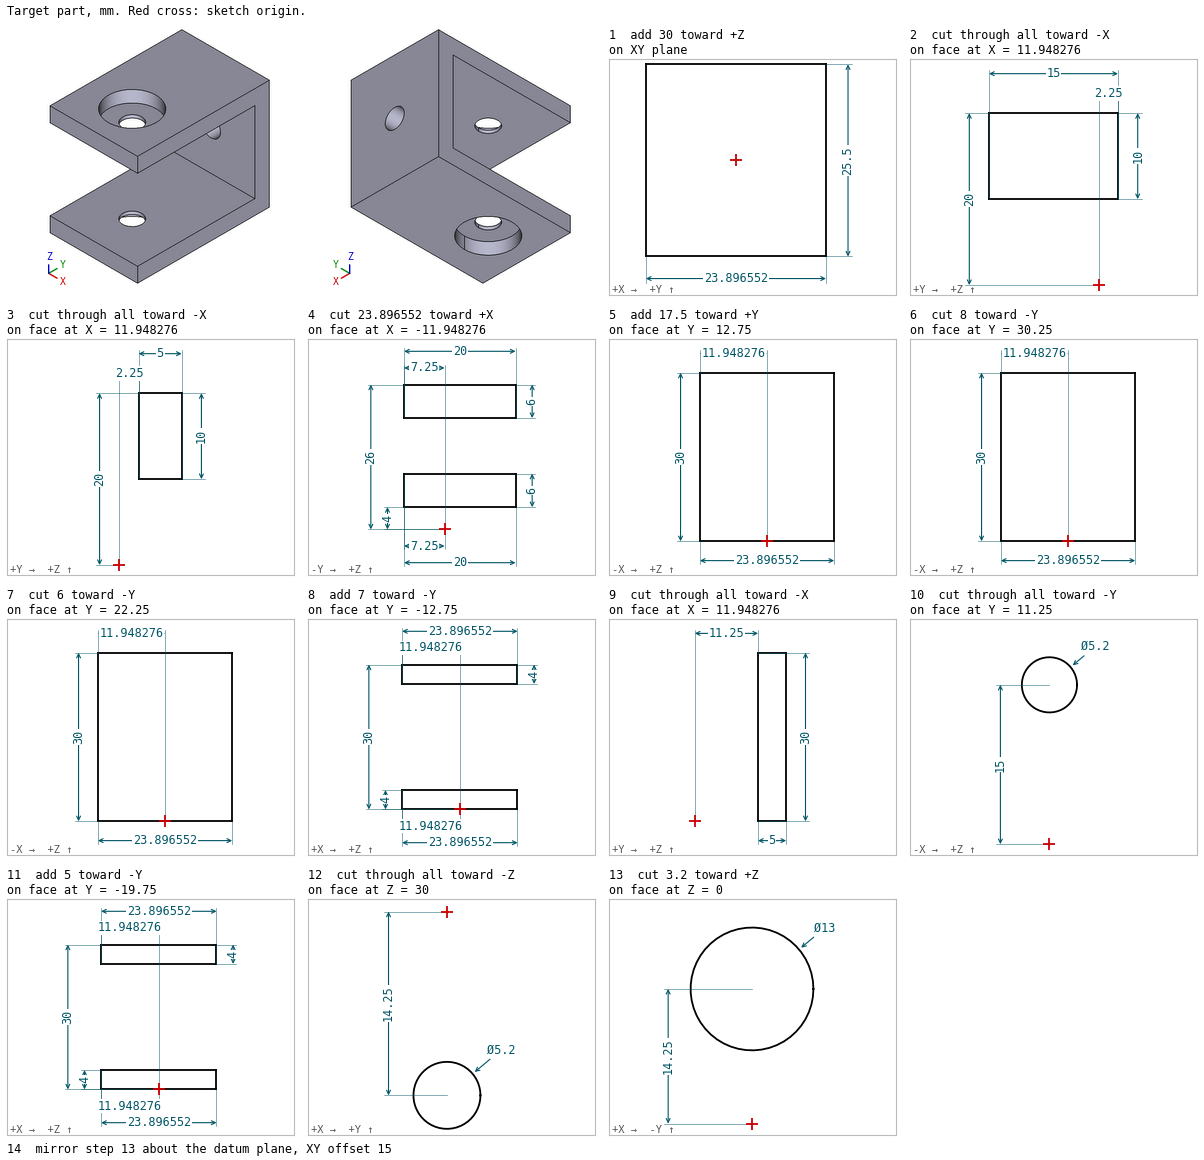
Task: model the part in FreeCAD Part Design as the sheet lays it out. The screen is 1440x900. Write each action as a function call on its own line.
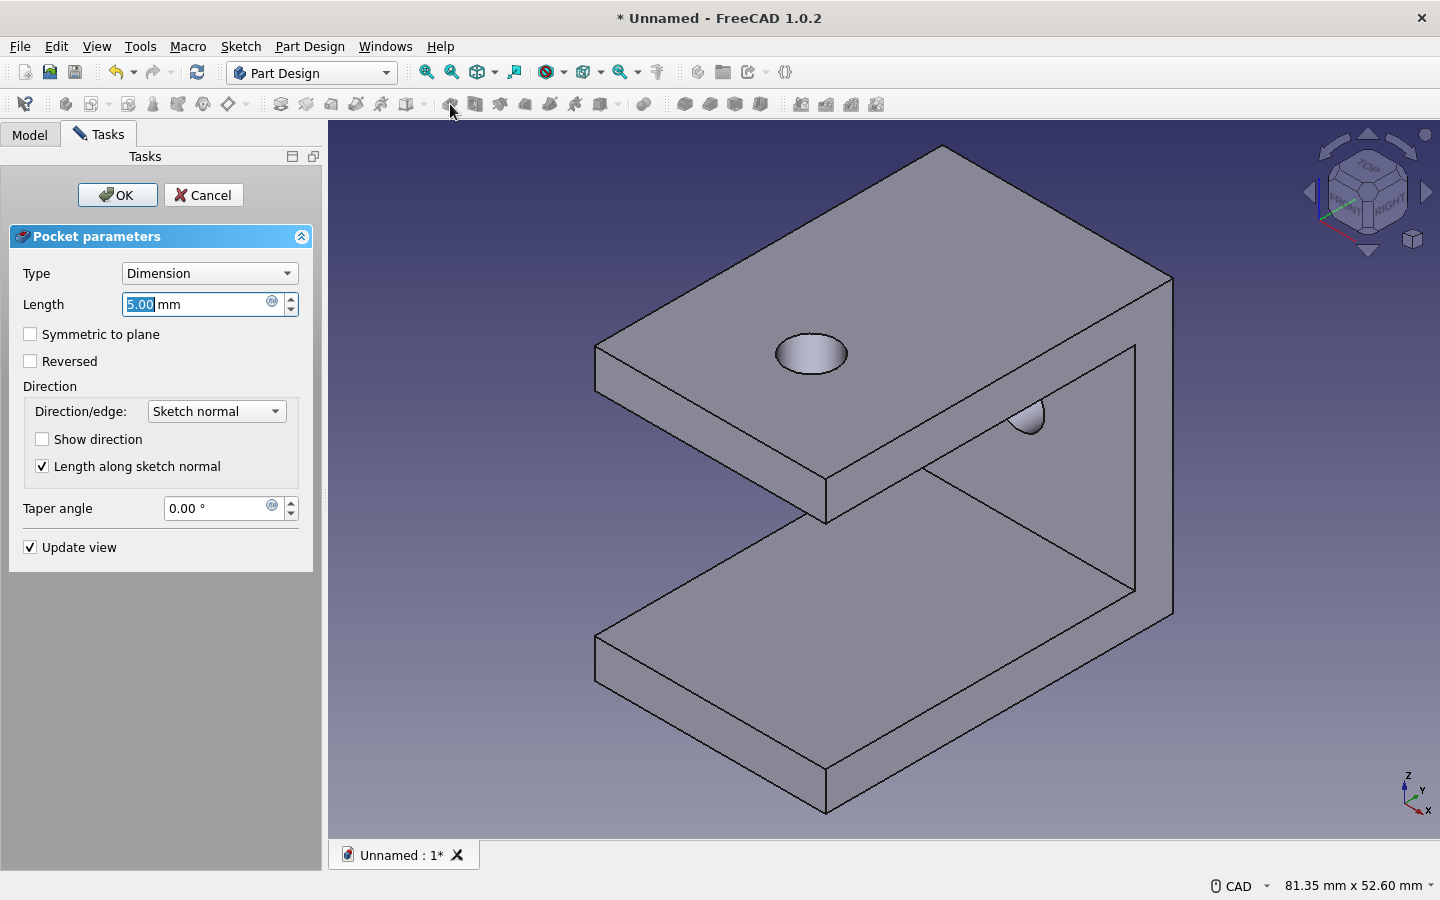
click(210, 274)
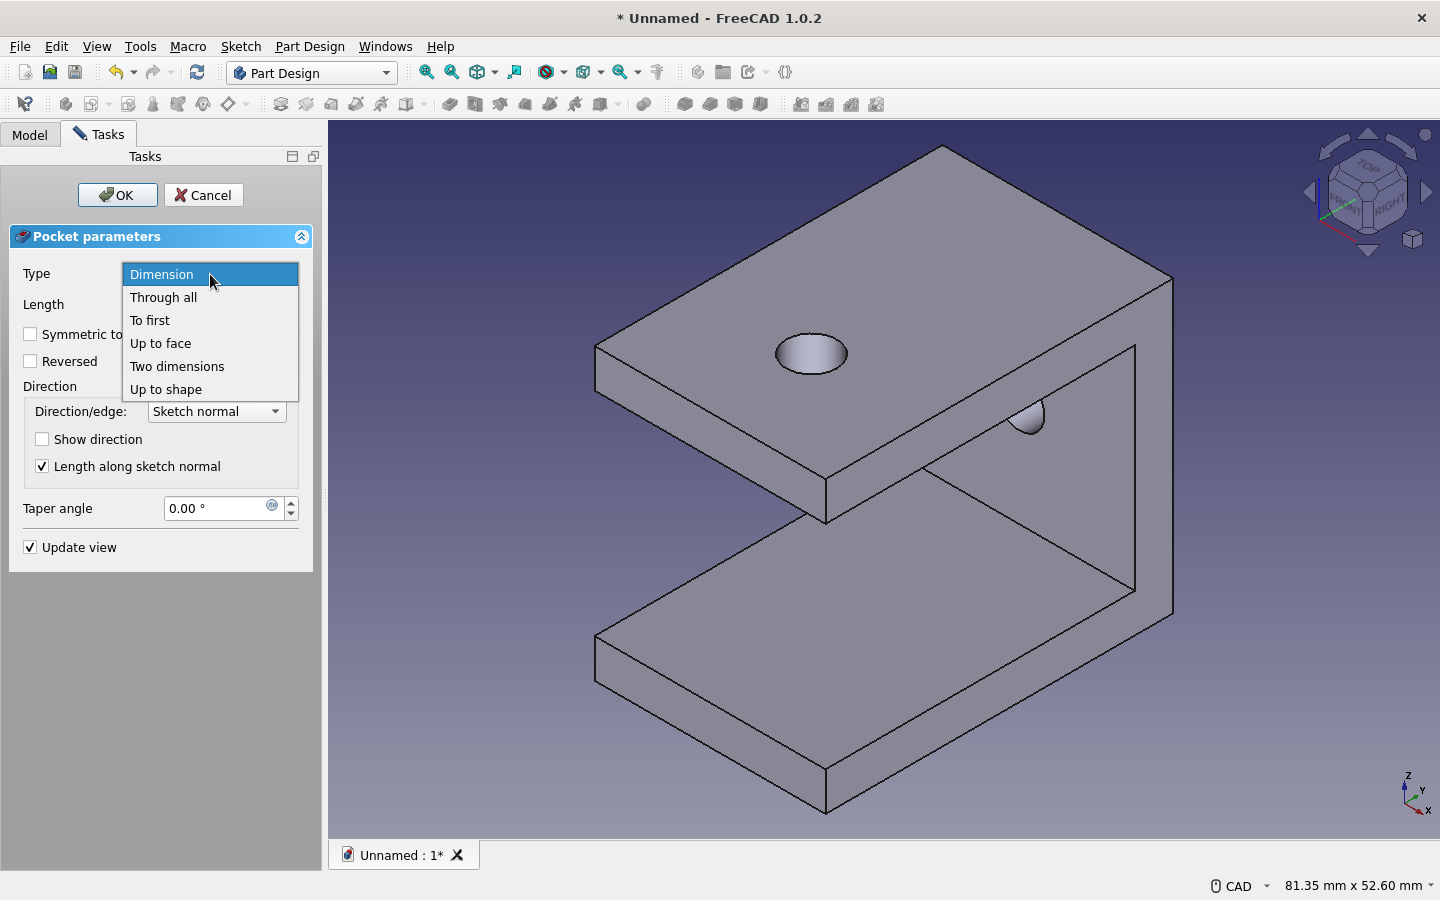
click(208, 298)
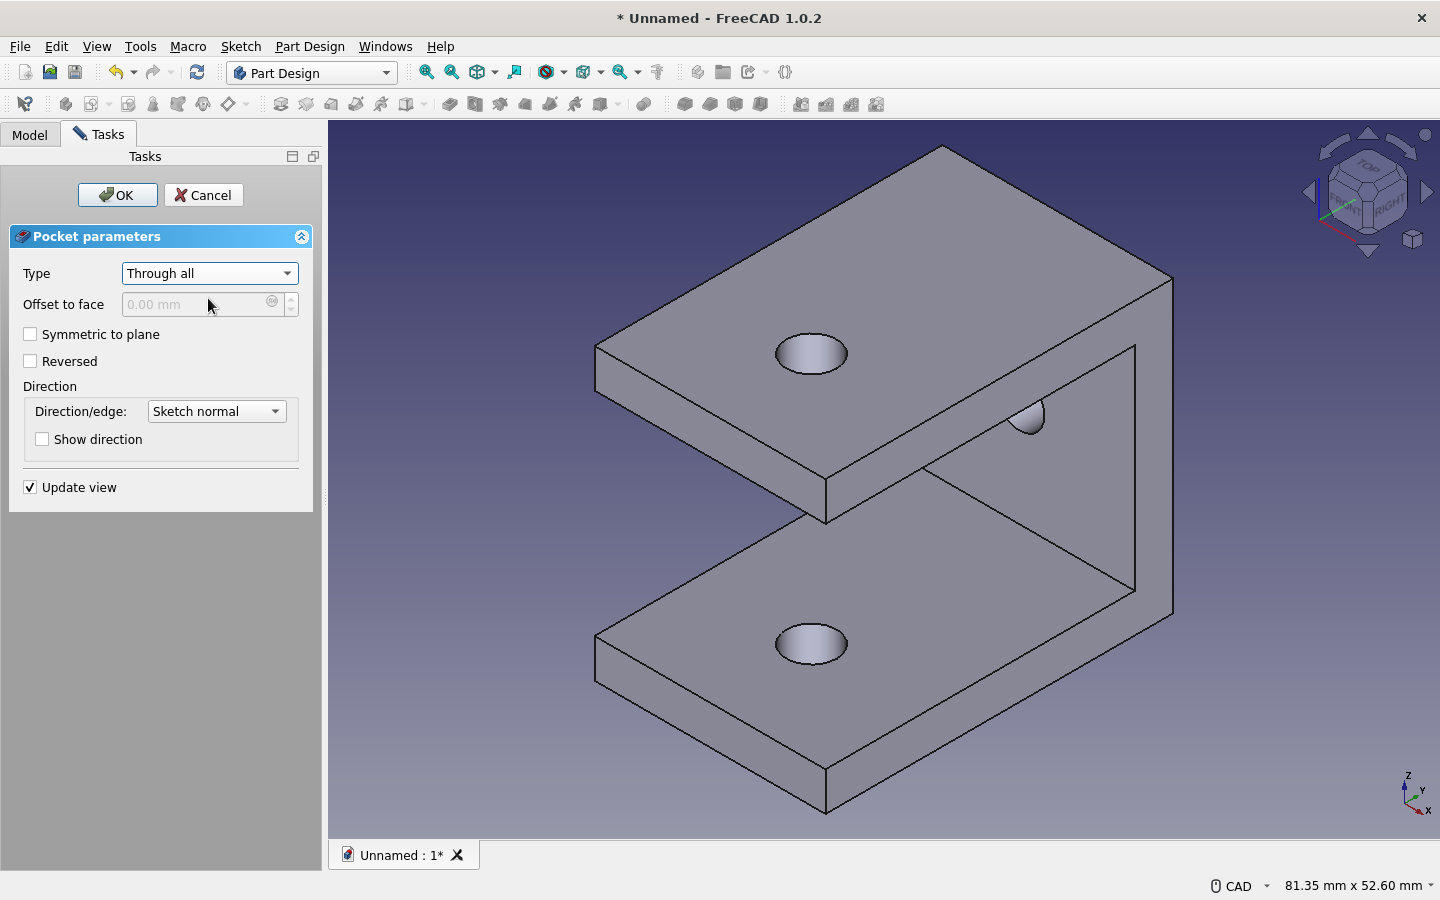
click(118, 195)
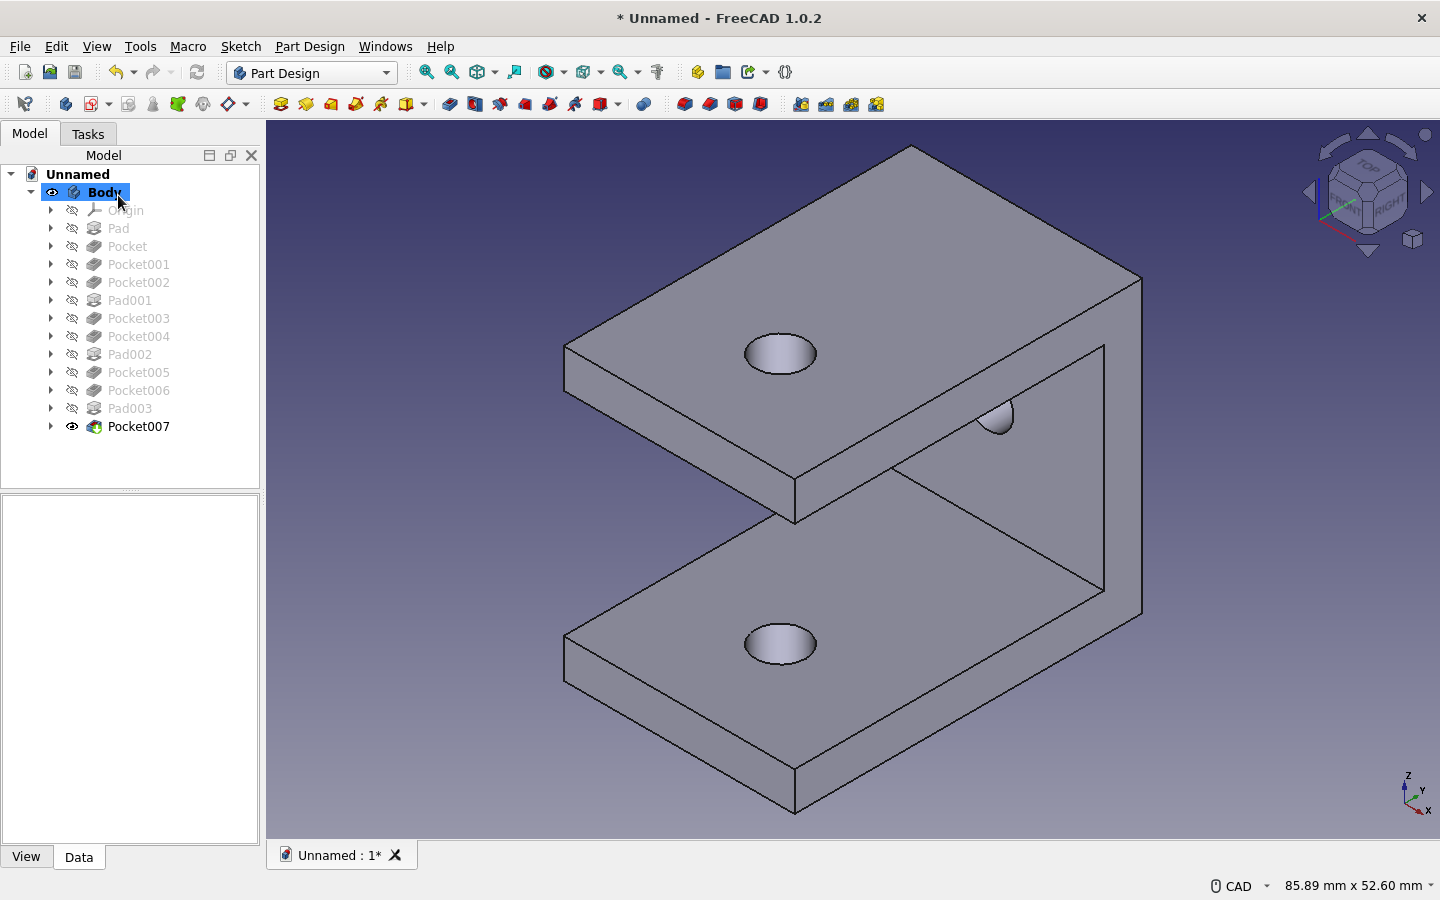
key(5)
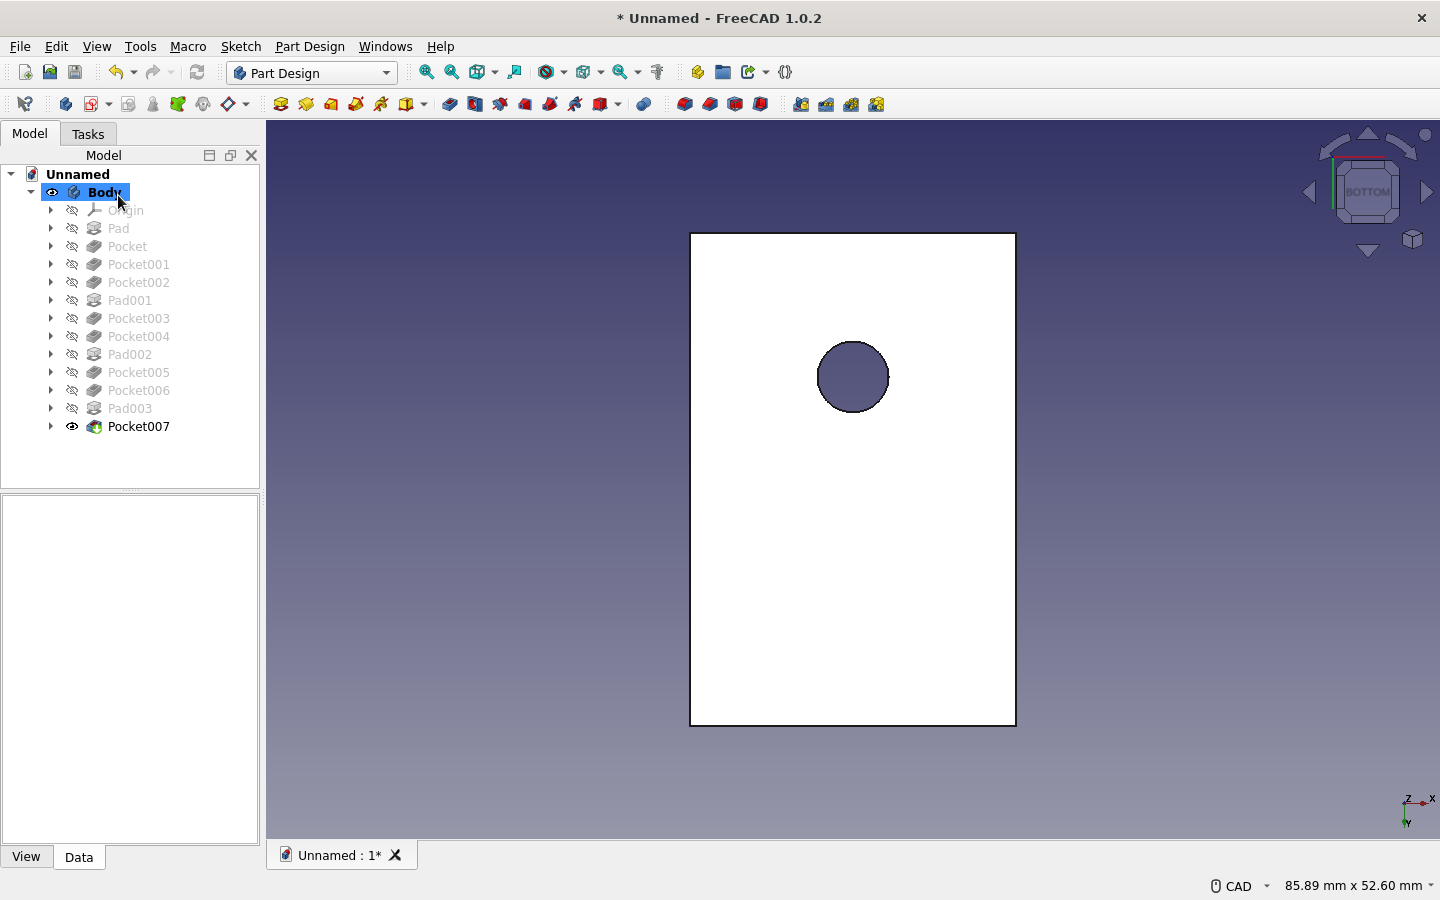
click(853, 549)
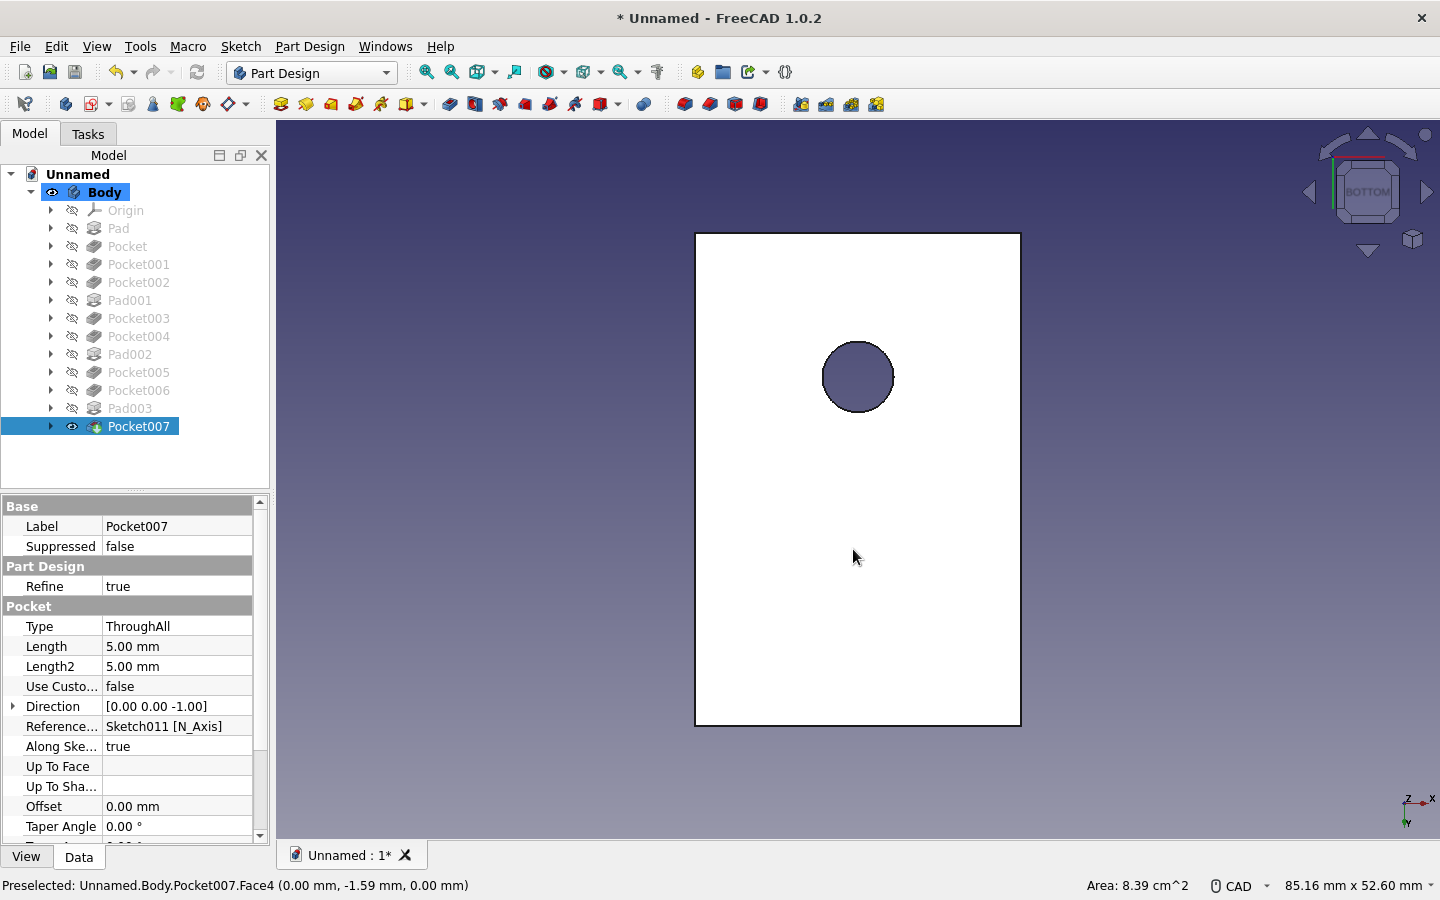
click(90, 104)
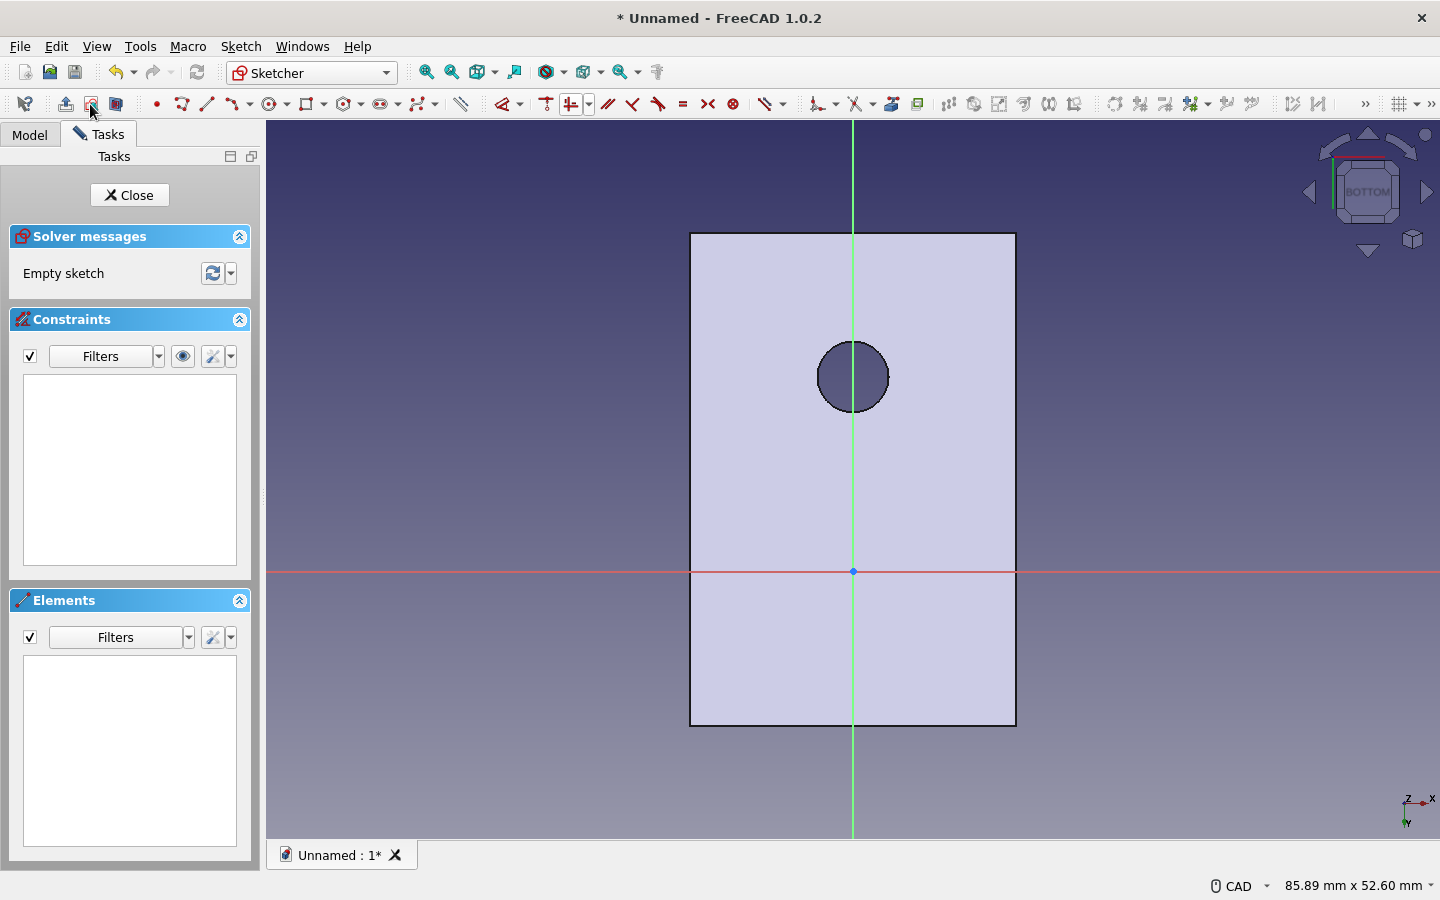
scroll(936, 370, up, 3)